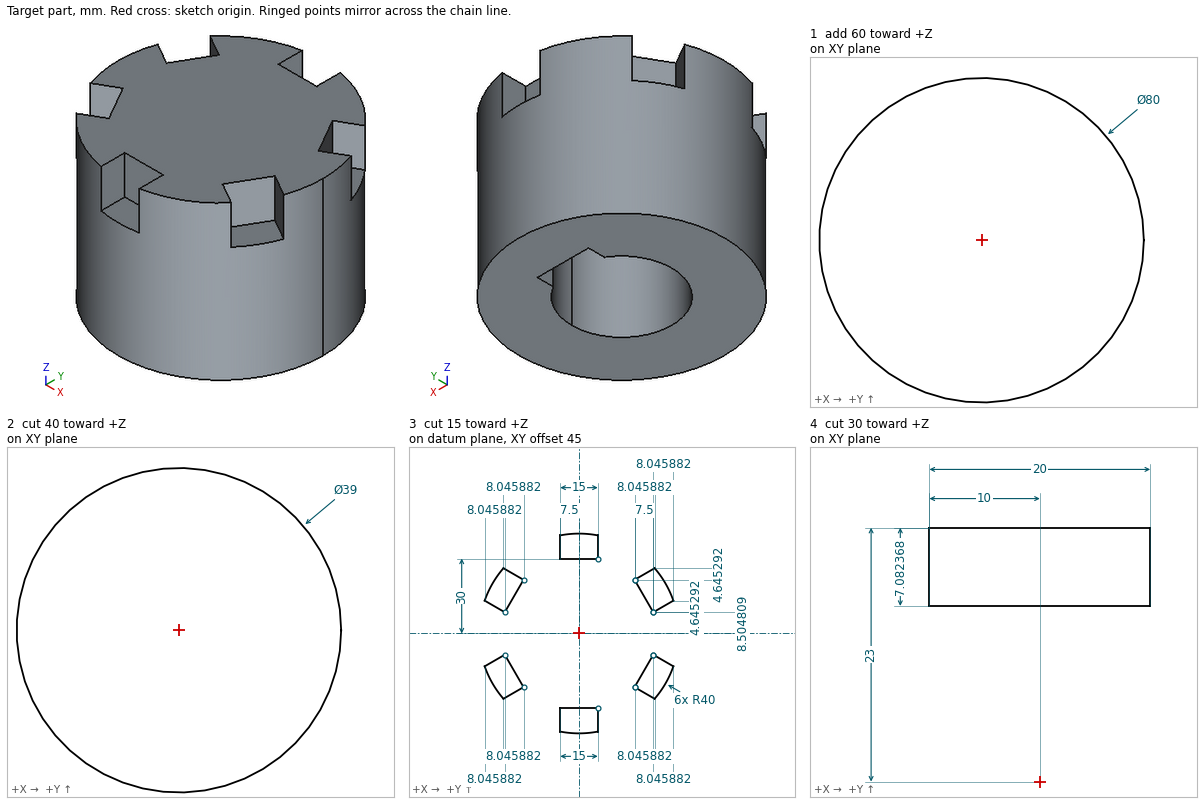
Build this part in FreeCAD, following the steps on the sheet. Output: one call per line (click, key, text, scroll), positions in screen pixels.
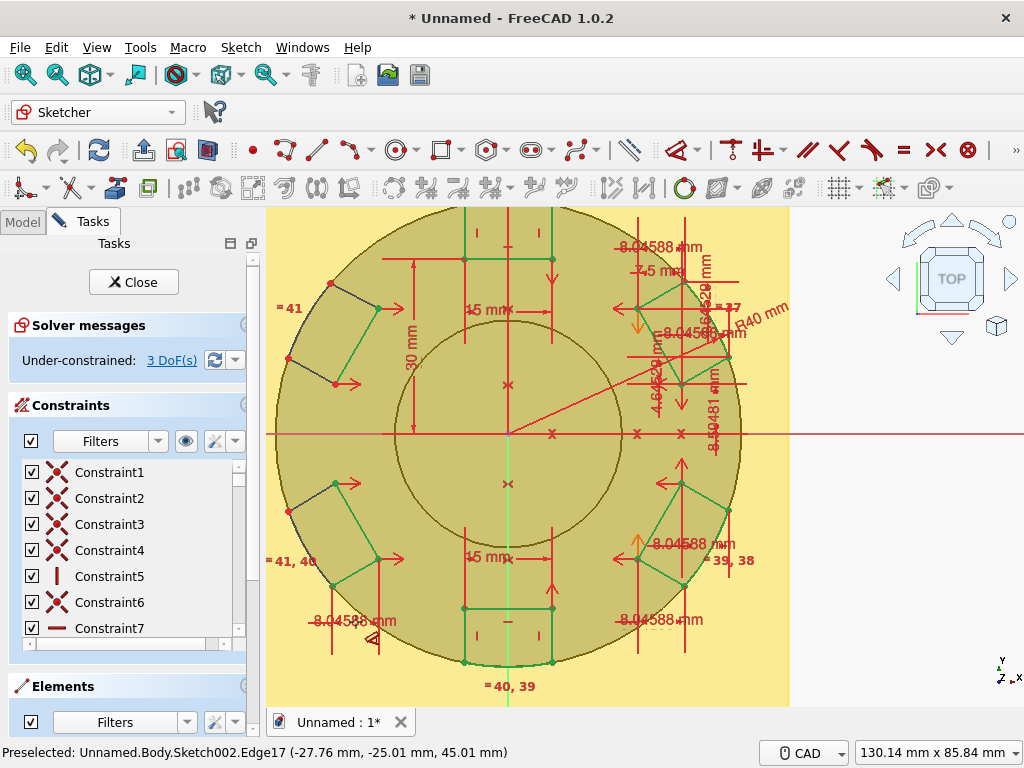
click(321, 492)
click(324, 546)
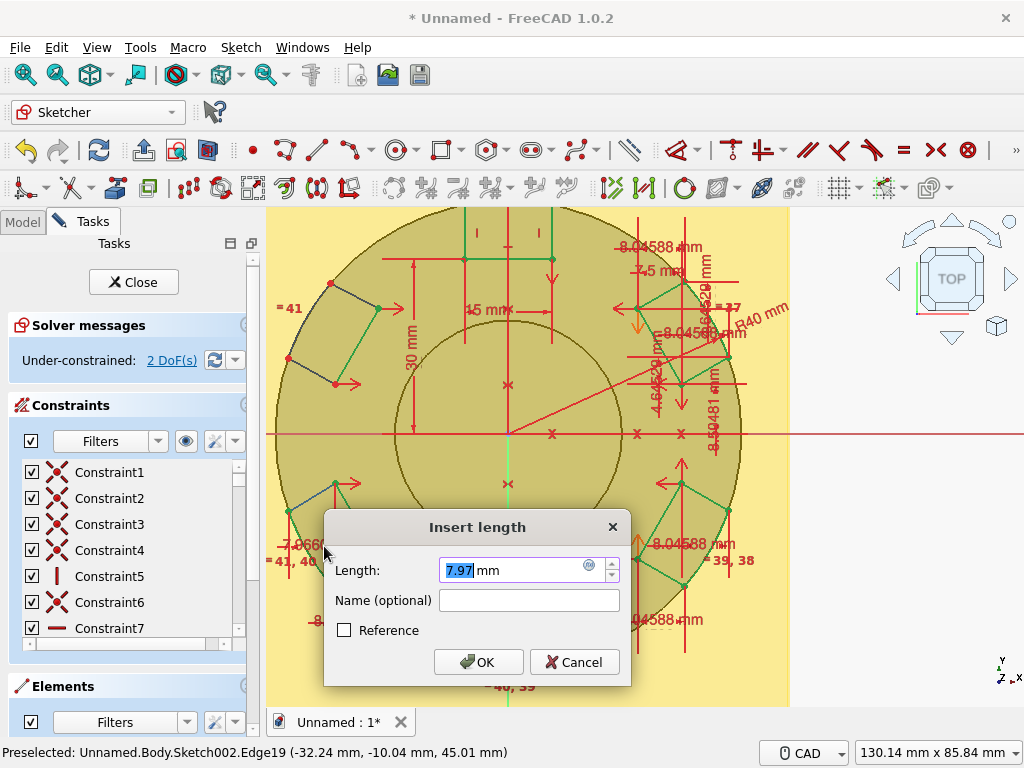
text(8.045882)
key(Return)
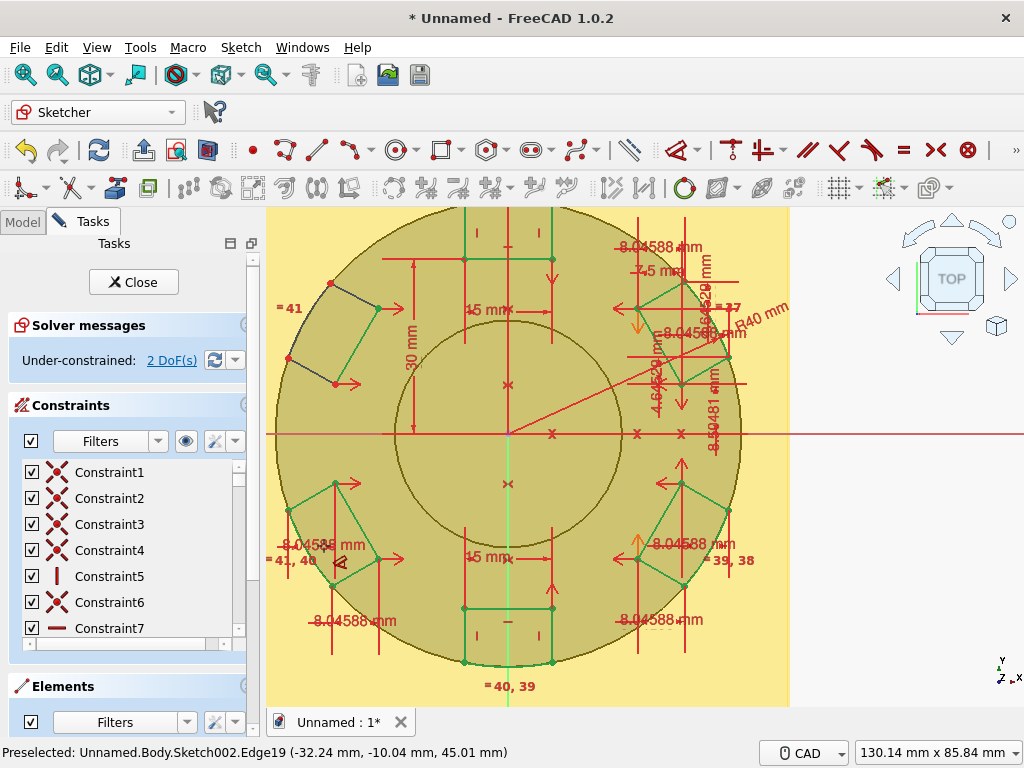
click(302, 366)
click(324, 324)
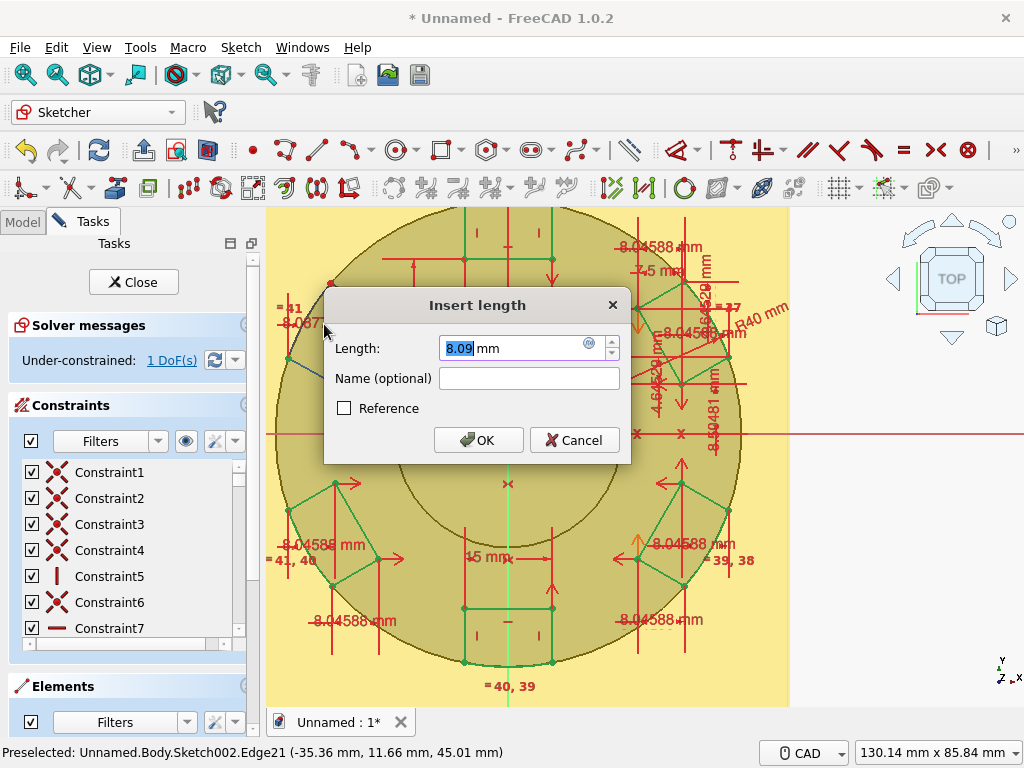
text(8.045882)
key(Return)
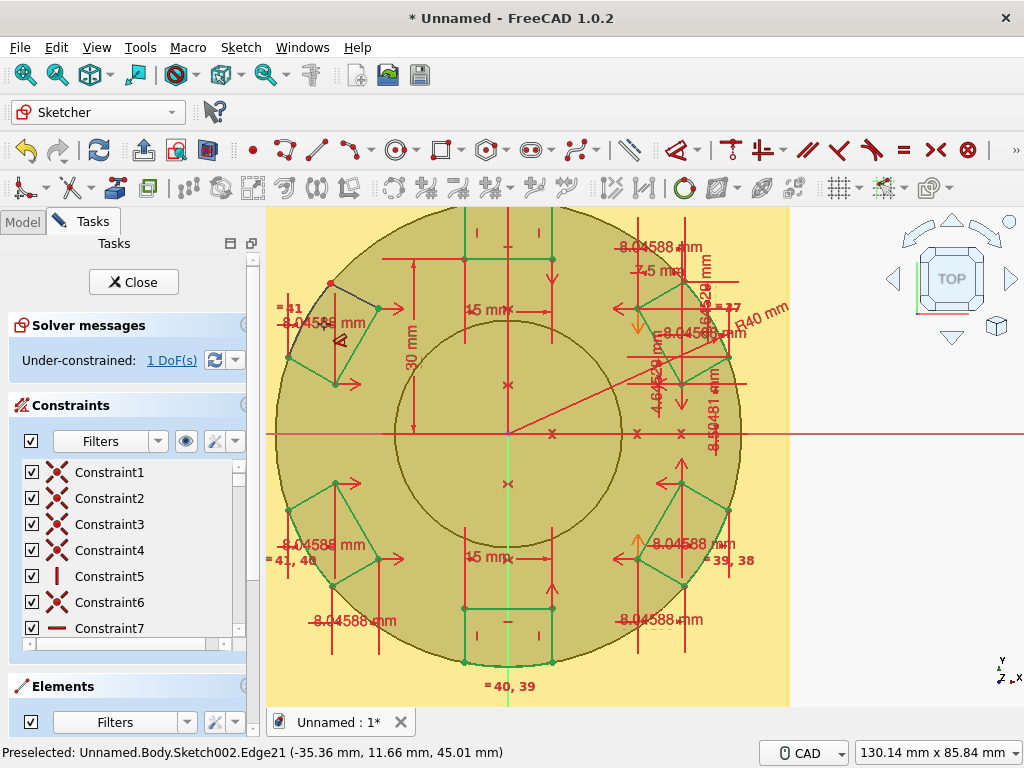
click(364, 301)
click(355, 249)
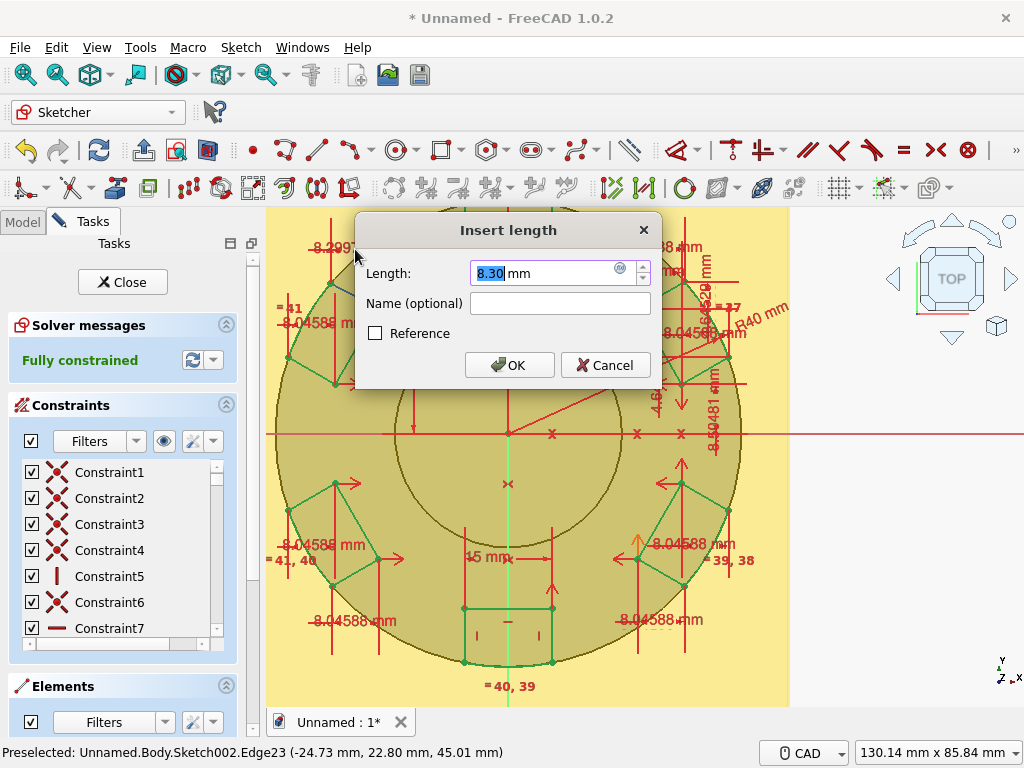
text(8.045882)
key(Return)
key(Escape)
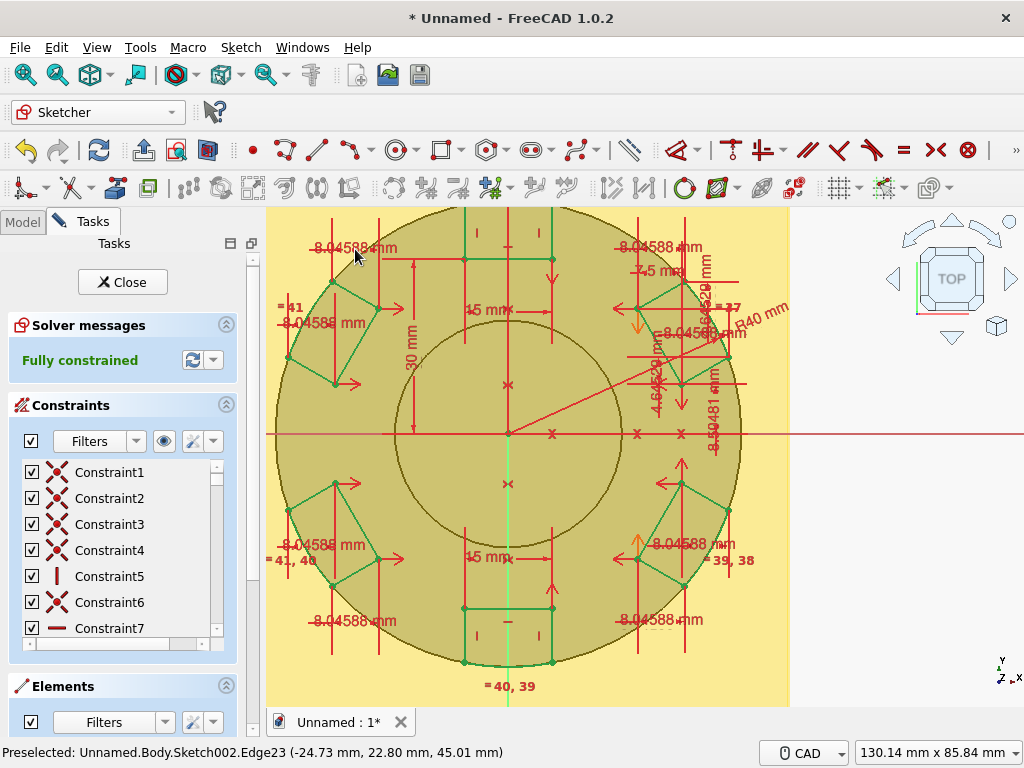
click(123, 282)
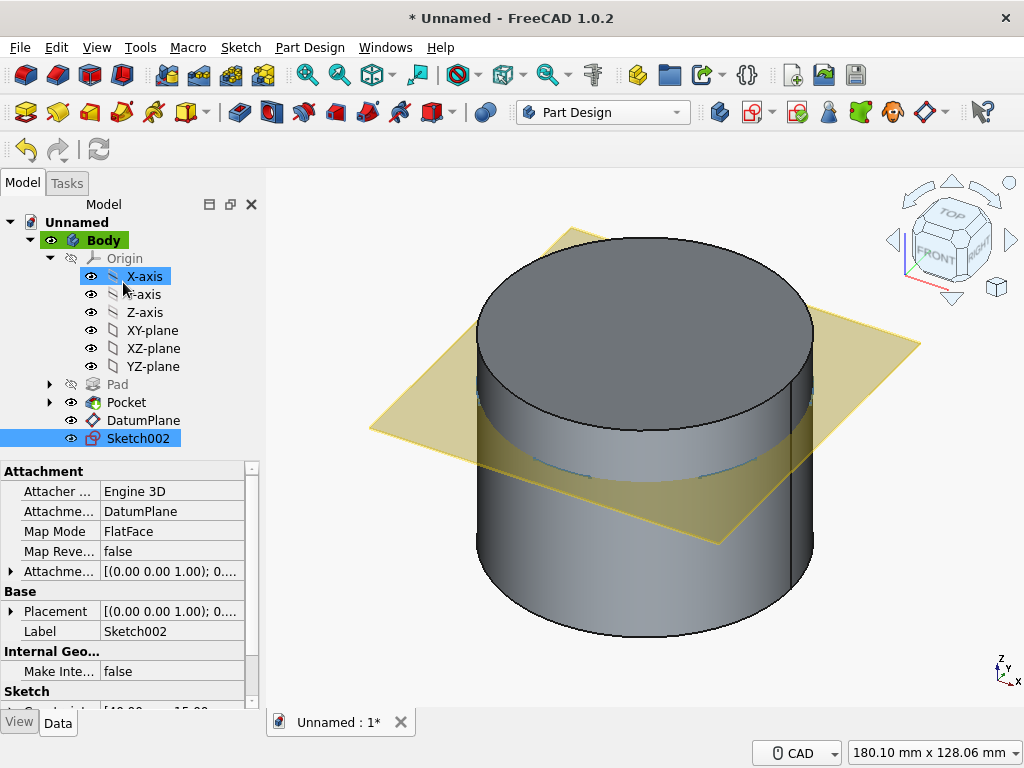
click(240, 112)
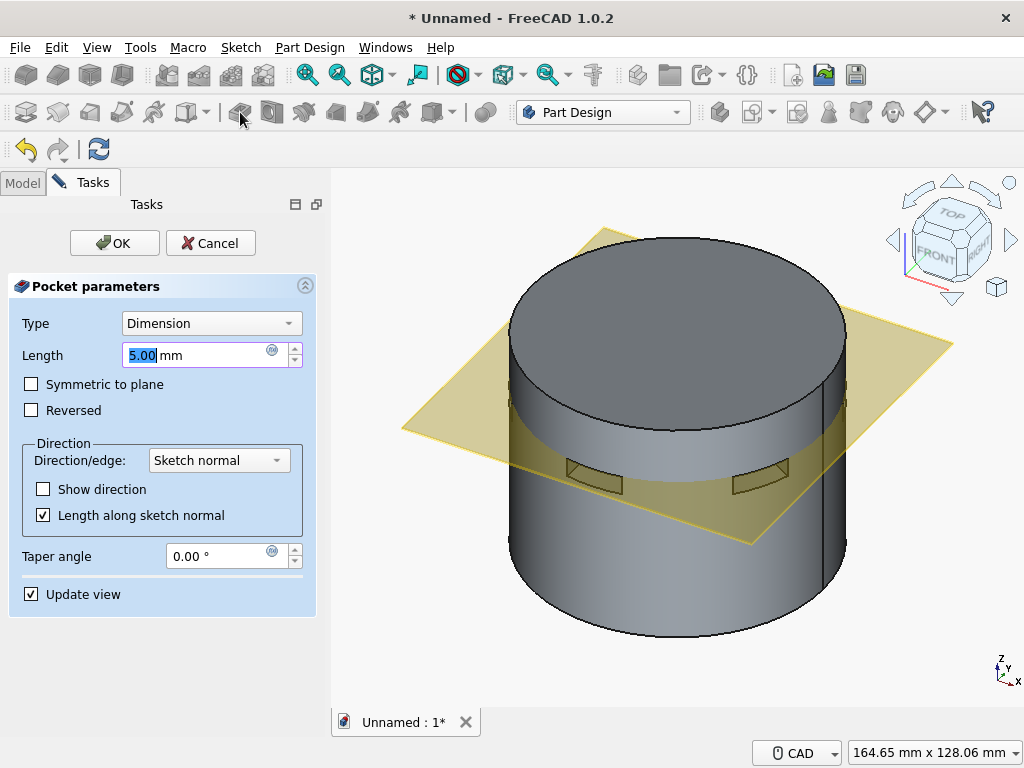
text(15)
key(Tab)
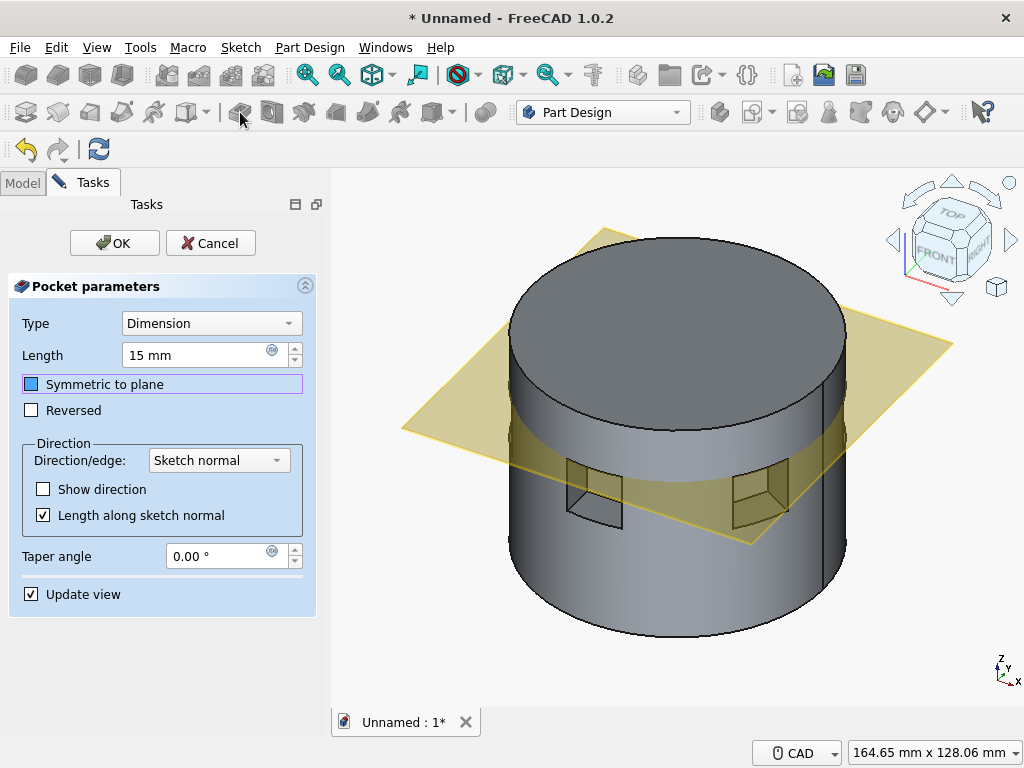
click(30, 410)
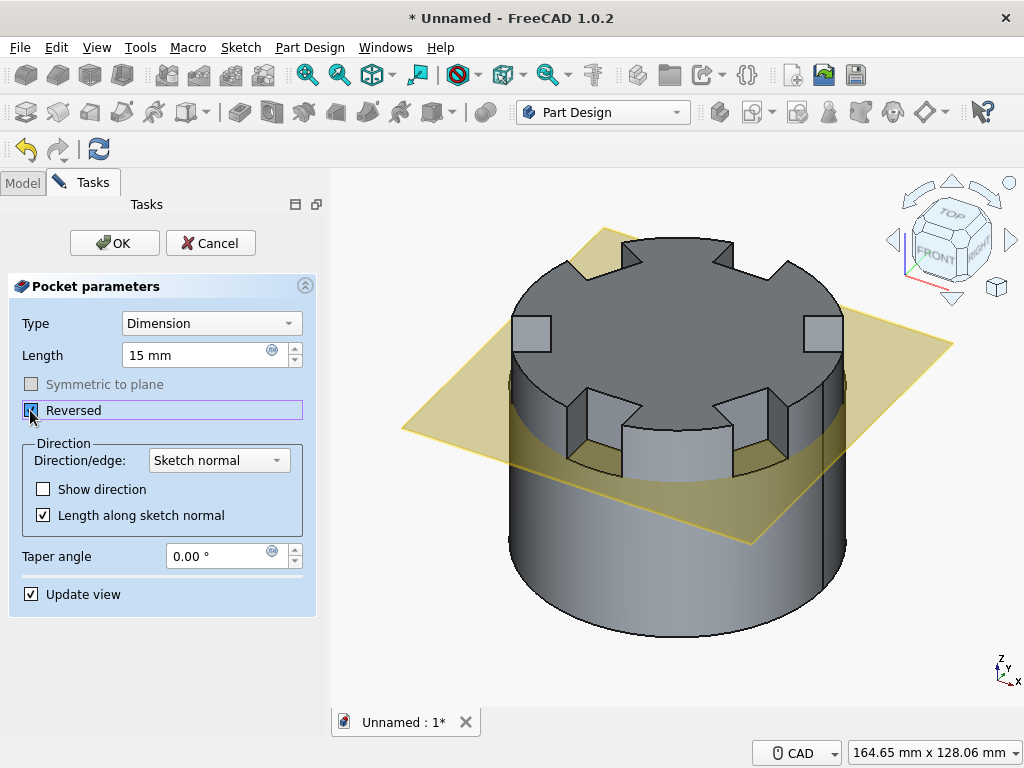
click(115, 243)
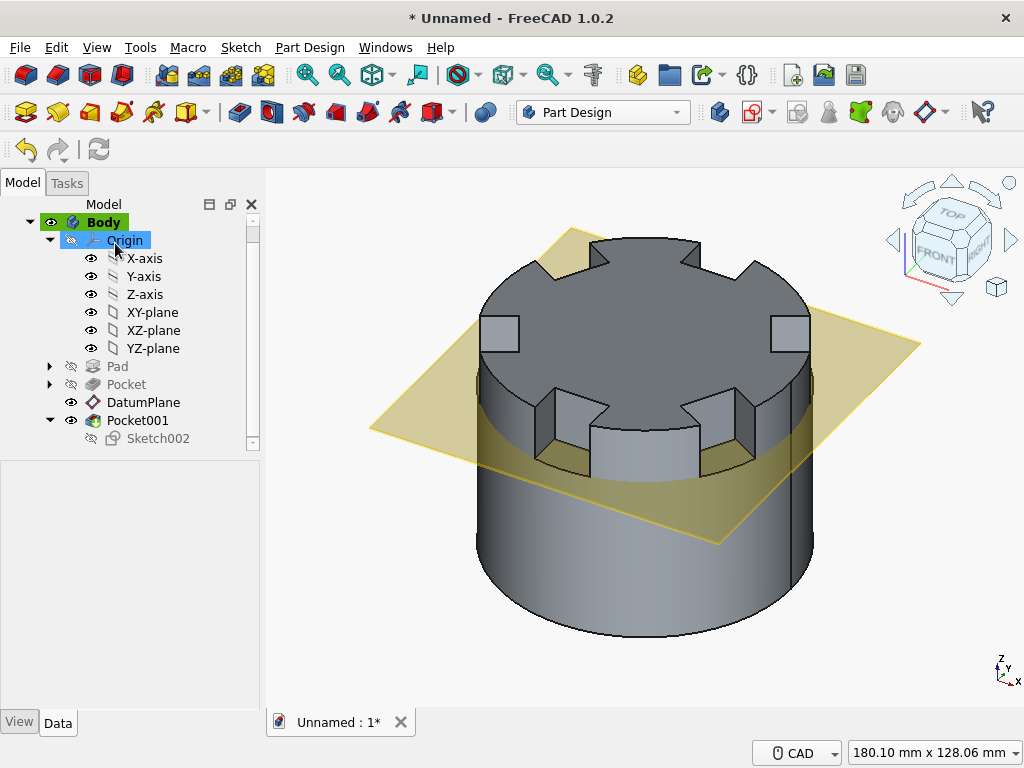
click(116, 402)
key(space)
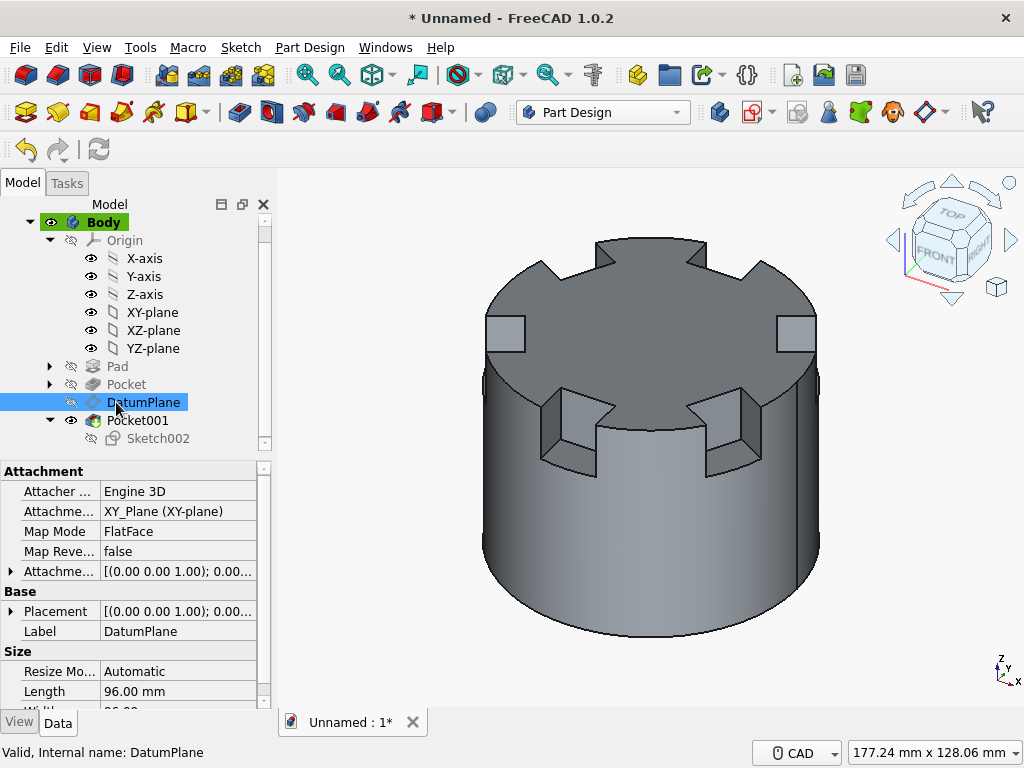
click(318, 667)